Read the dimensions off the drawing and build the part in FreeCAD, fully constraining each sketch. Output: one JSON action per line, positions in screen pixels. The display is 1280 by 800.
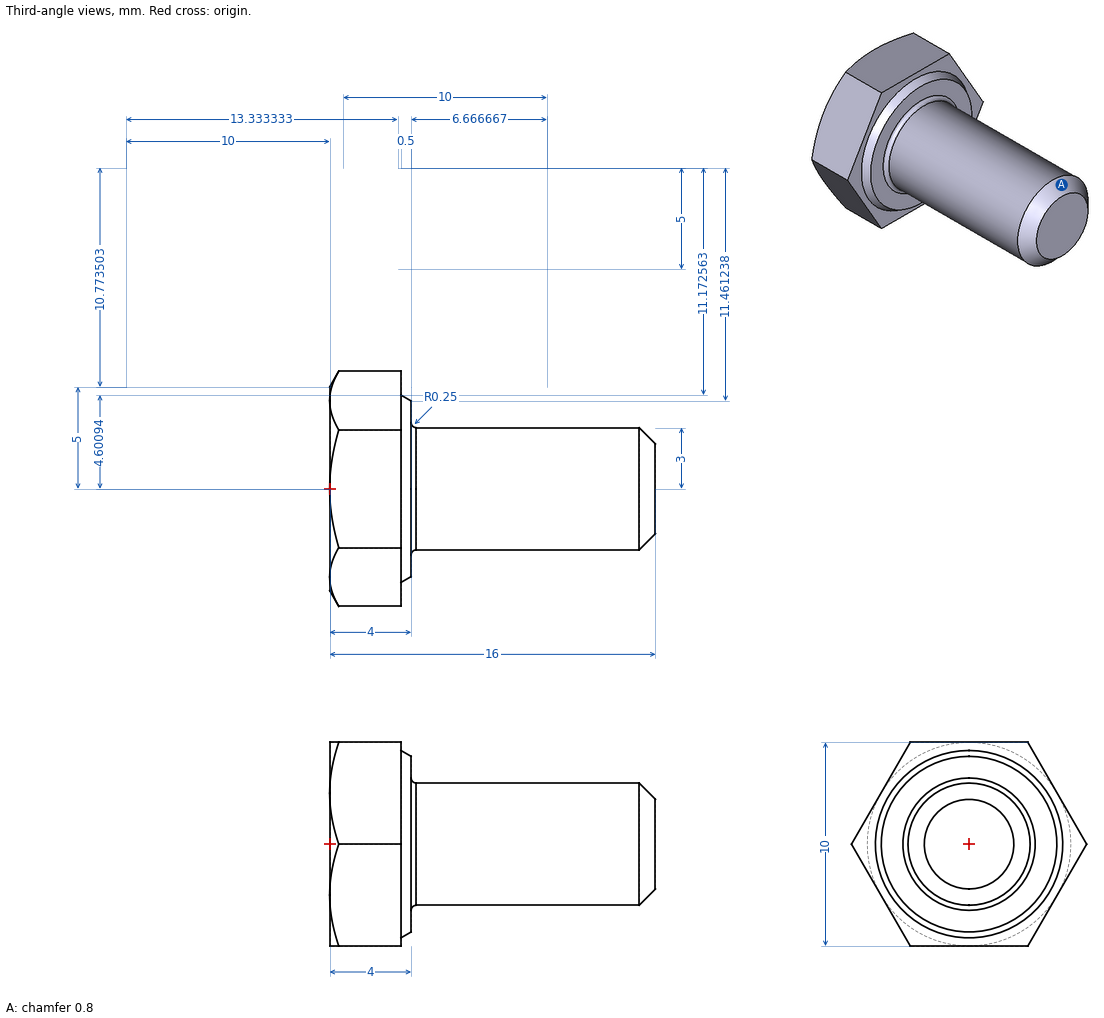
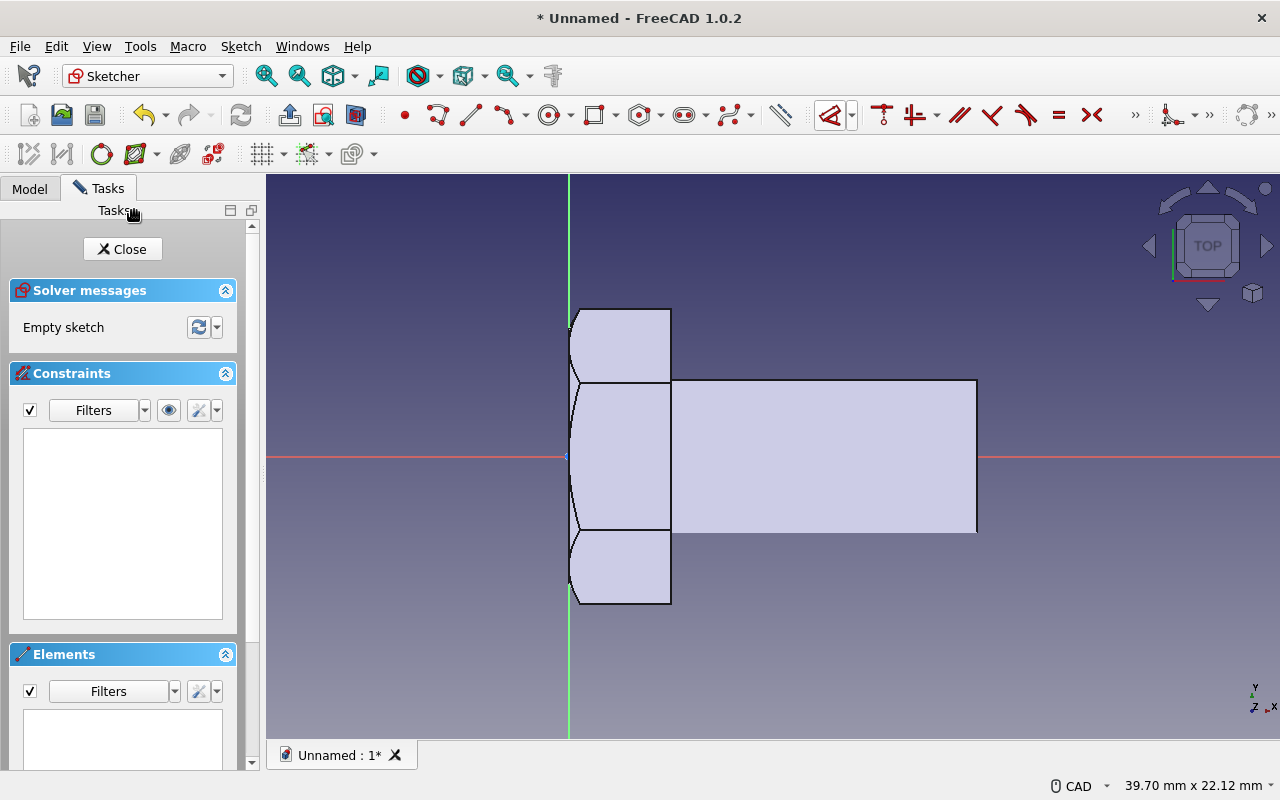
{"action": "left_click", "coordinate": [356, 116]}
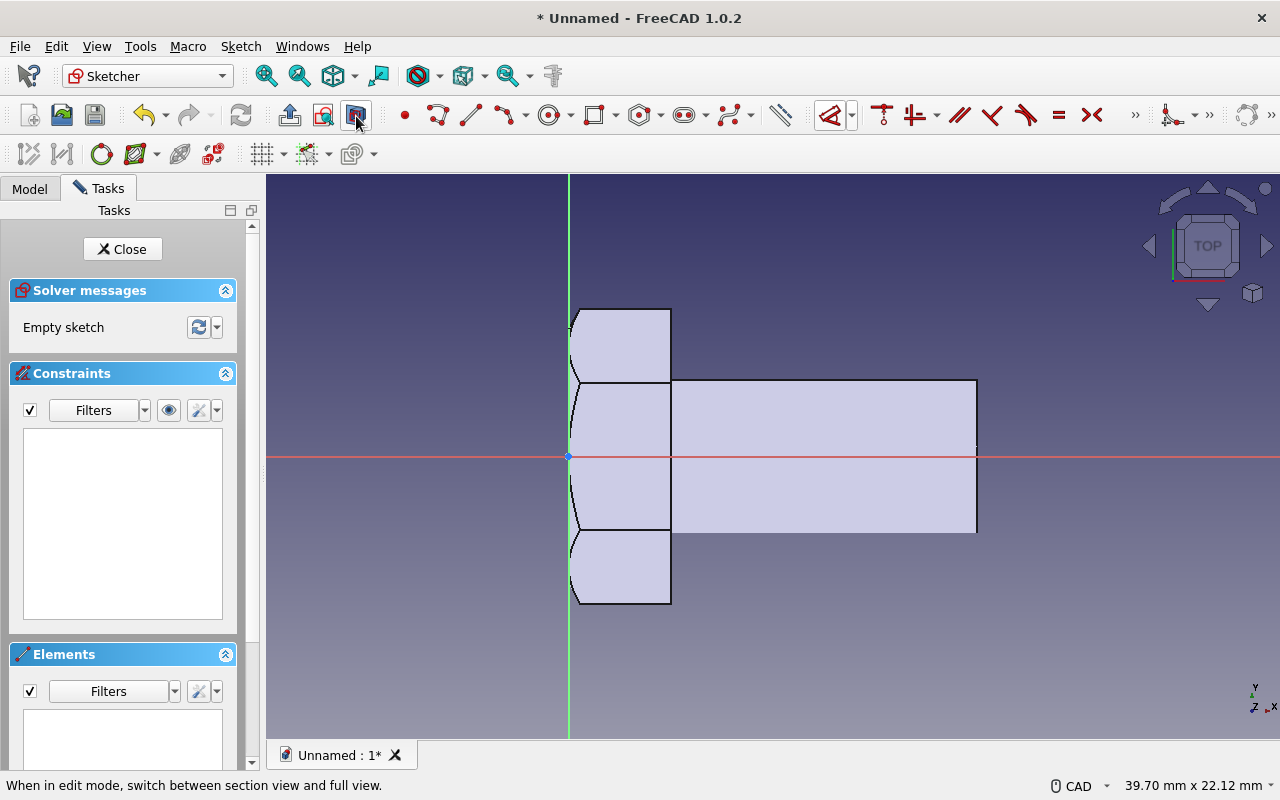
{"action": "scroll", "coordinate": [704, 711], "scroll_direction": "down", "scroll_amount": 2}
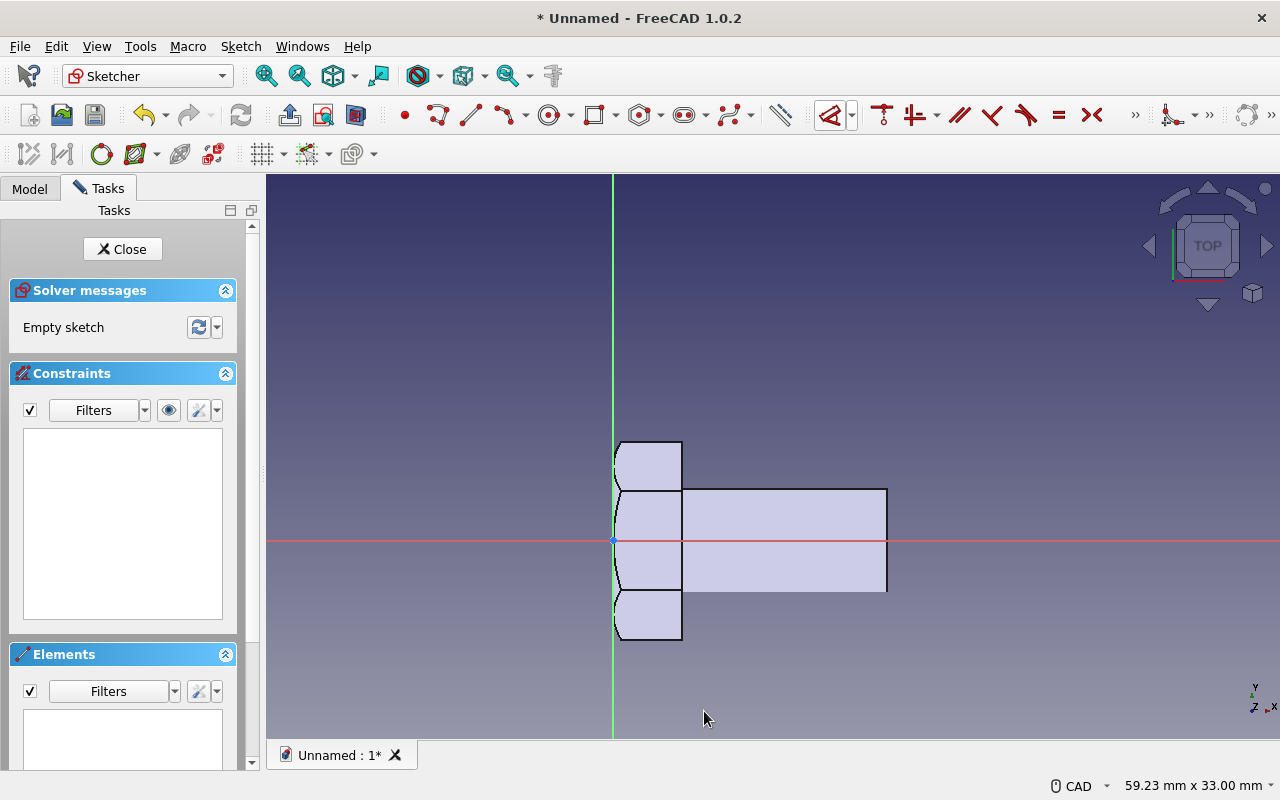
{"action": "left_click", "coordinate": [438, 116]}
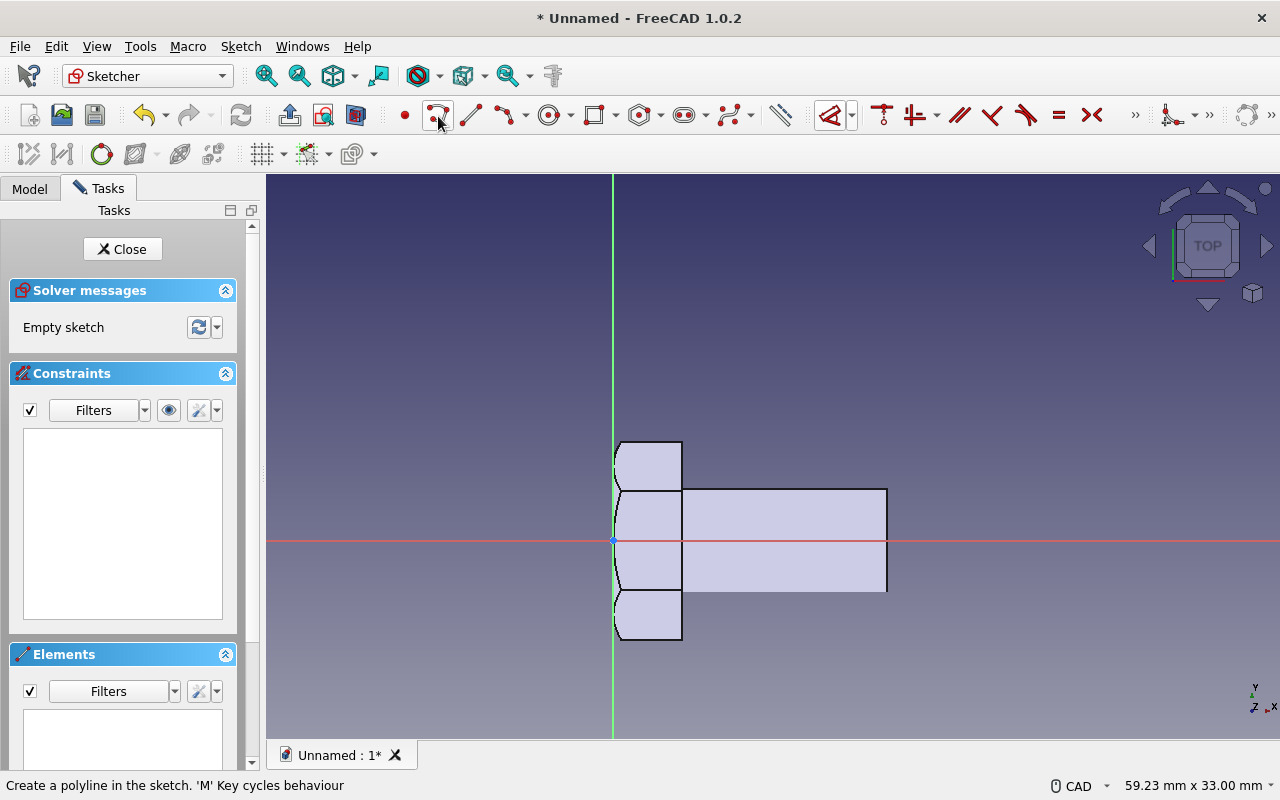
{"action": "left_click", "coordinate": [682, 455]}
{"action": "left_click", "coordinate": [796, 455]}
{"action": "left_click", "coordinate": [796, 271]}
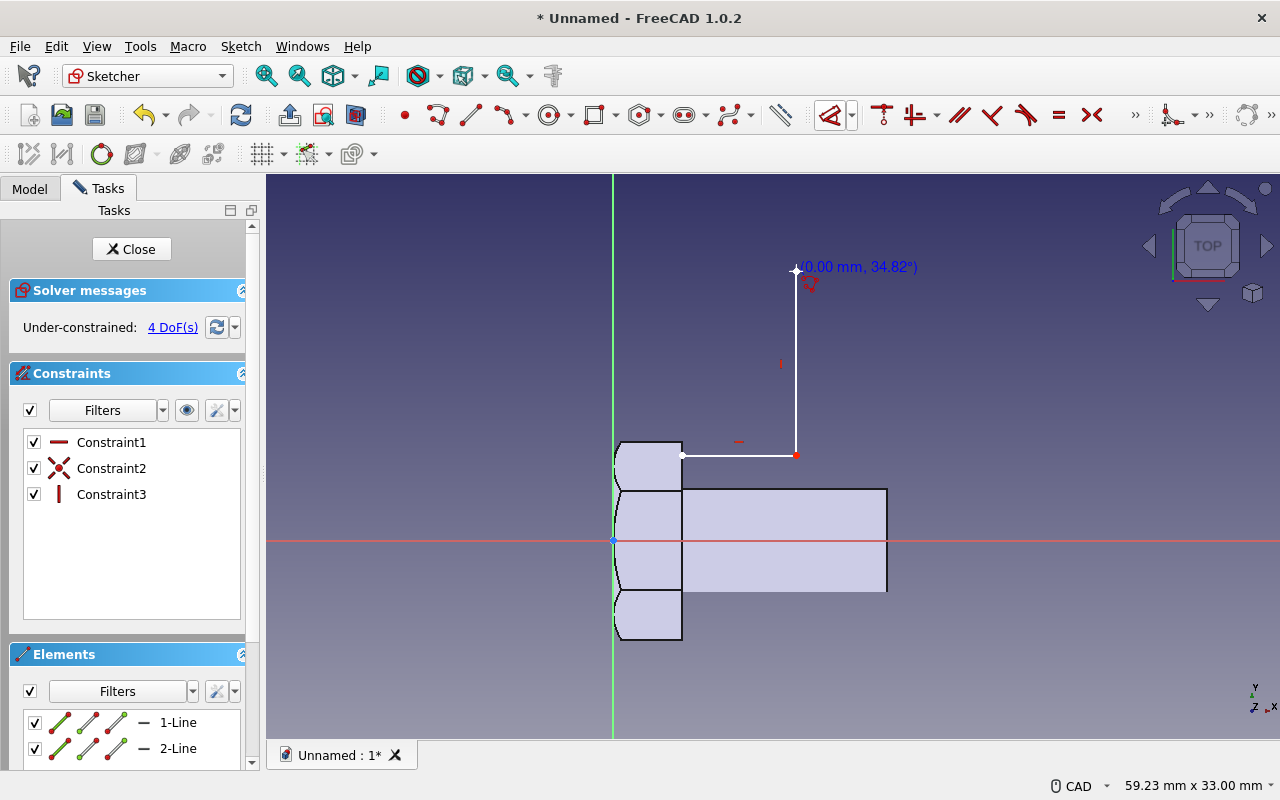
{"action": "scroll", "coordinate": [625, 271], "scroll_direction": "up", "scroll_amount": 2}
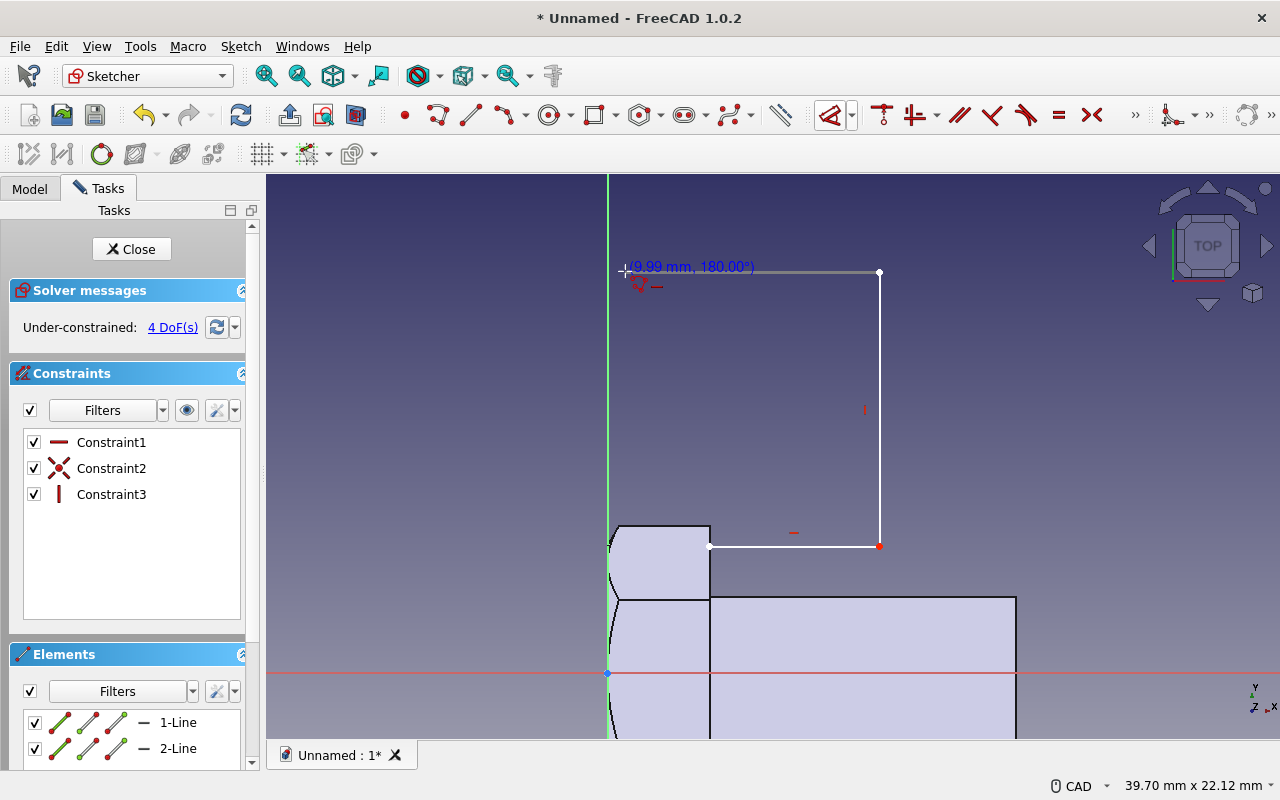
{"action": "left_click", "coordinate": [625, 271]}
{"action": "left_click", "coordinate": [625, 398]}
{"action": "left_click", "coordinate": [710, 547]}
{"action": "key", "text": "Escape"}
{"action": "key", "text": "Escape"}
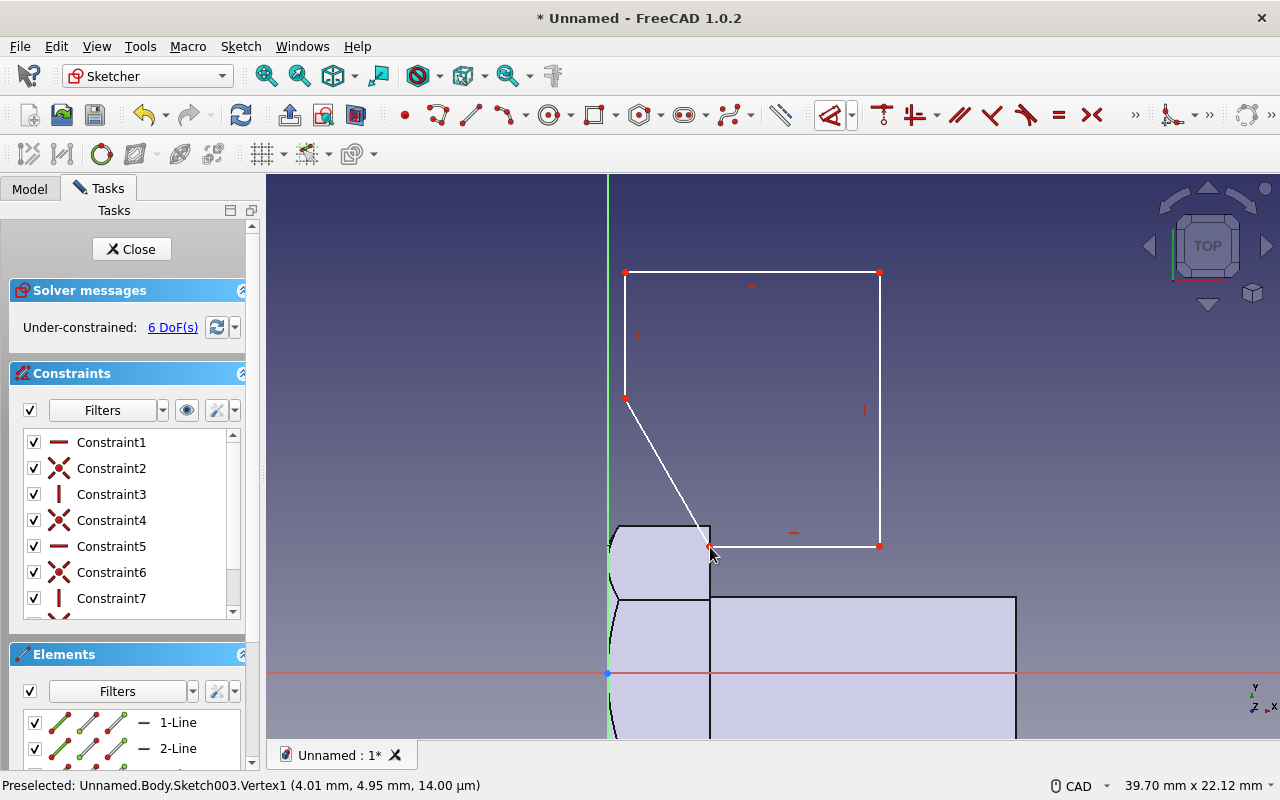
{"action": "left_click", "coordinate": [625, 310]}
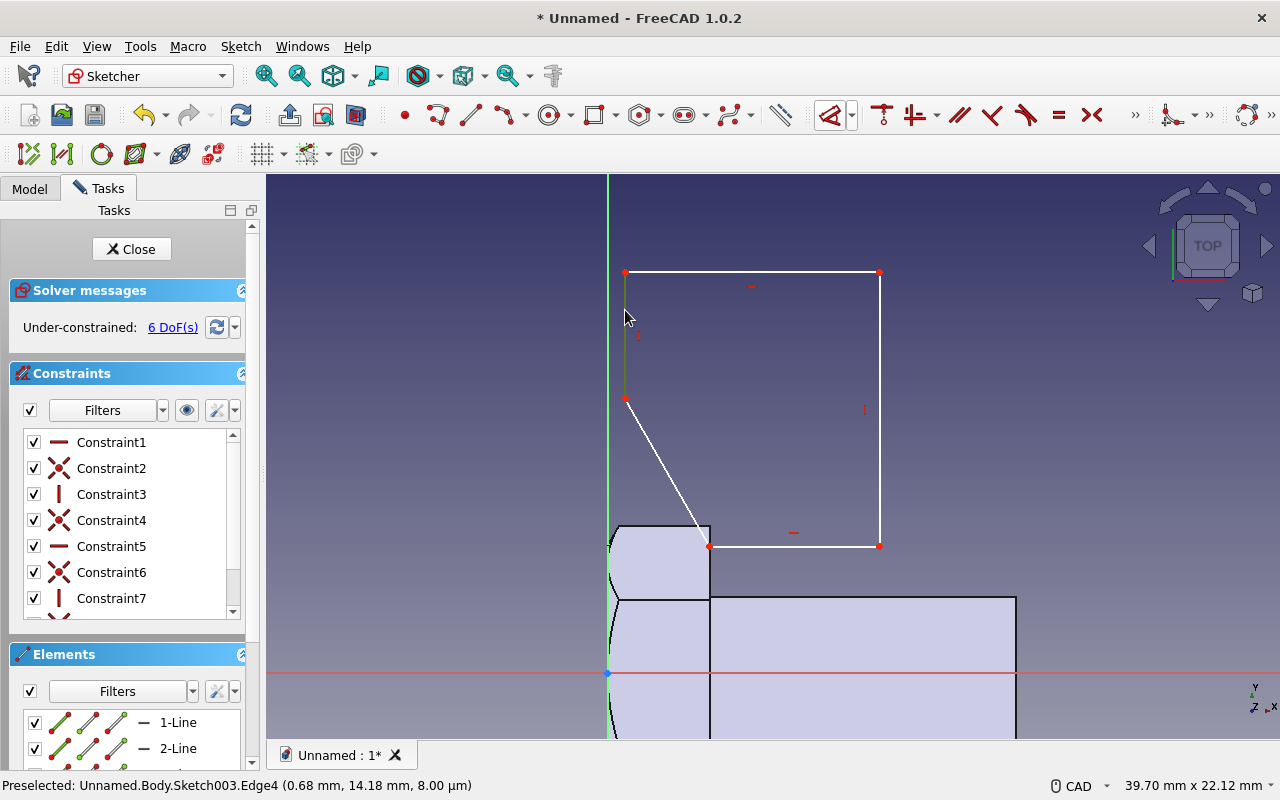
{"action": "left_click", "coordinate": [852, 116]}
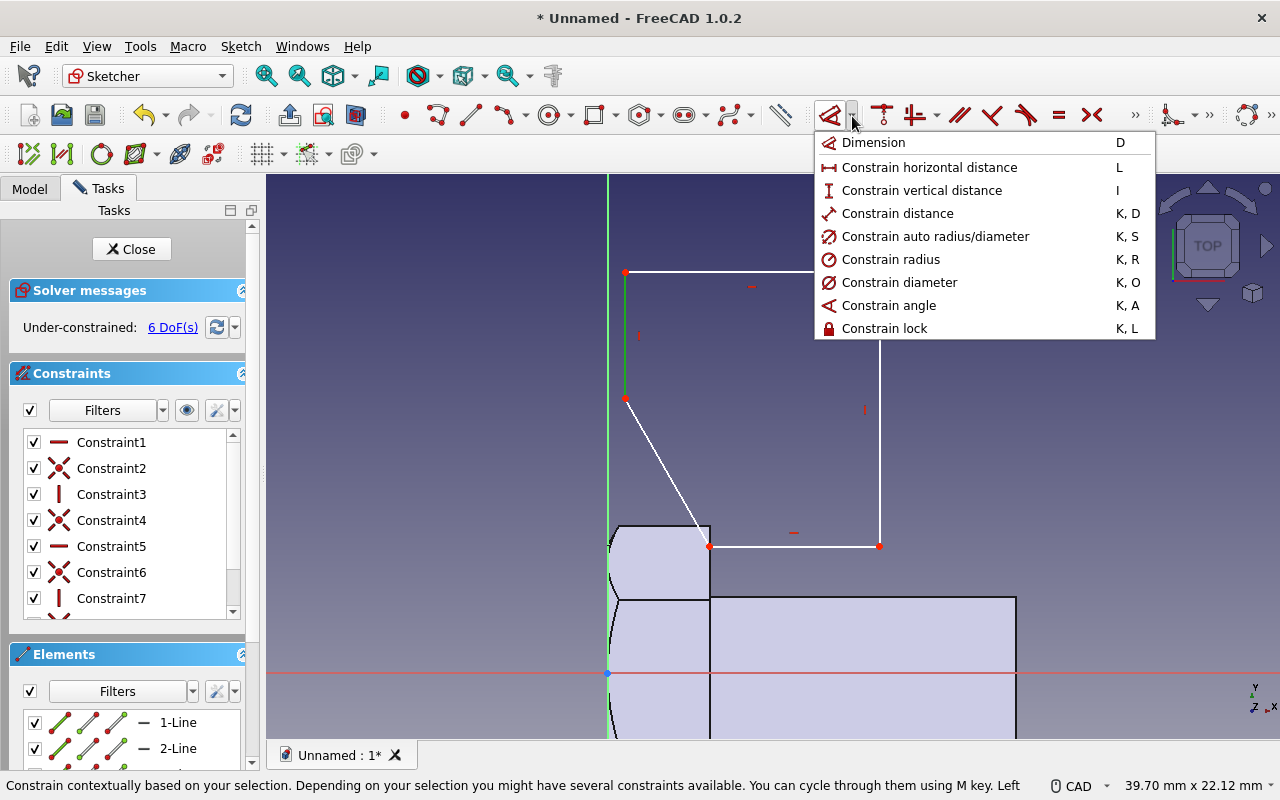
{"action": "left_click", "coordinate": [985, 190]}